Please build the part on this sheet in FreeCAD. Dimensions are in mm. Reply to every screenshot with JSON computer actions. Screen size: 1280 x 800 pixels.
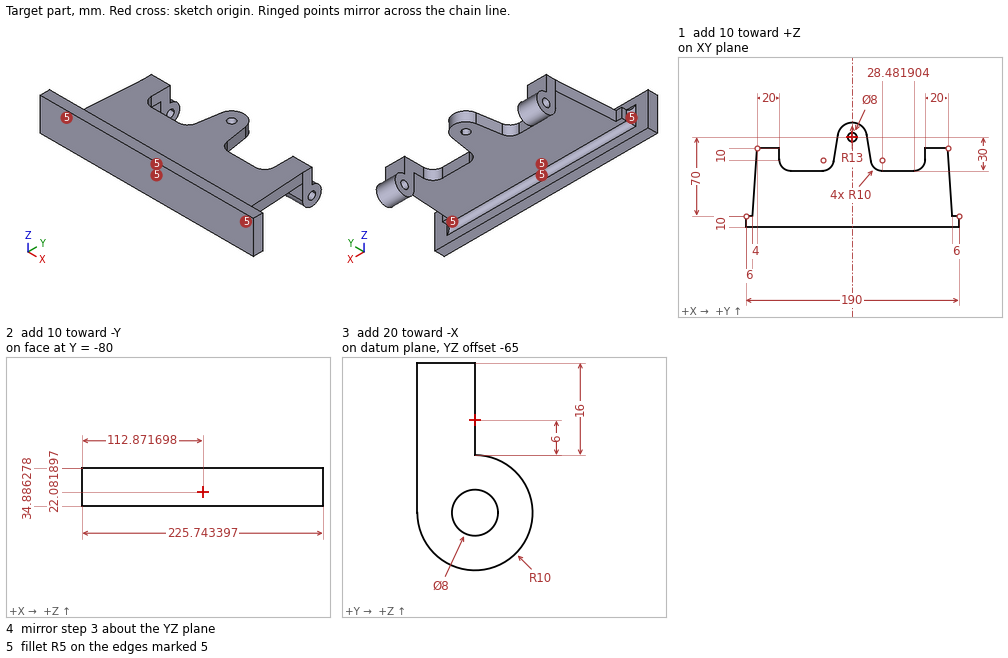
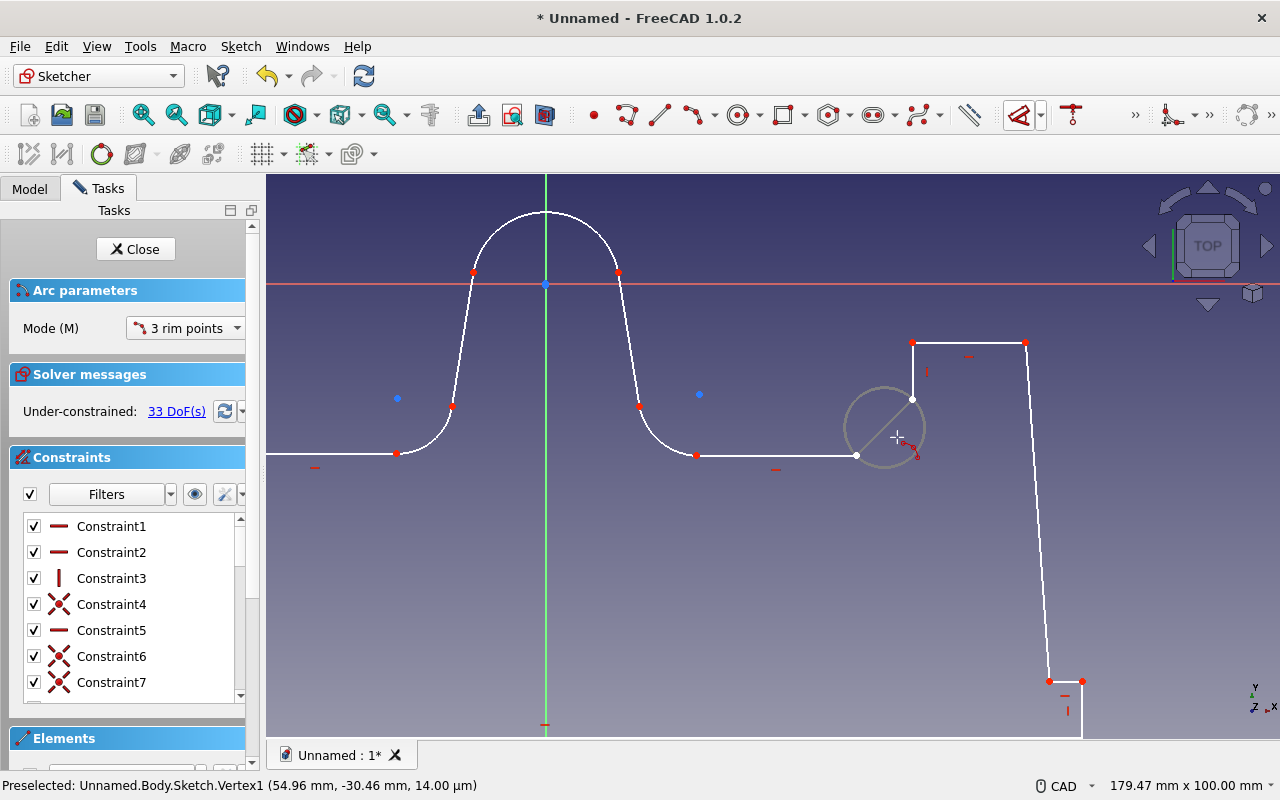
{"action": "left_click", "coordinate": [897, 437]}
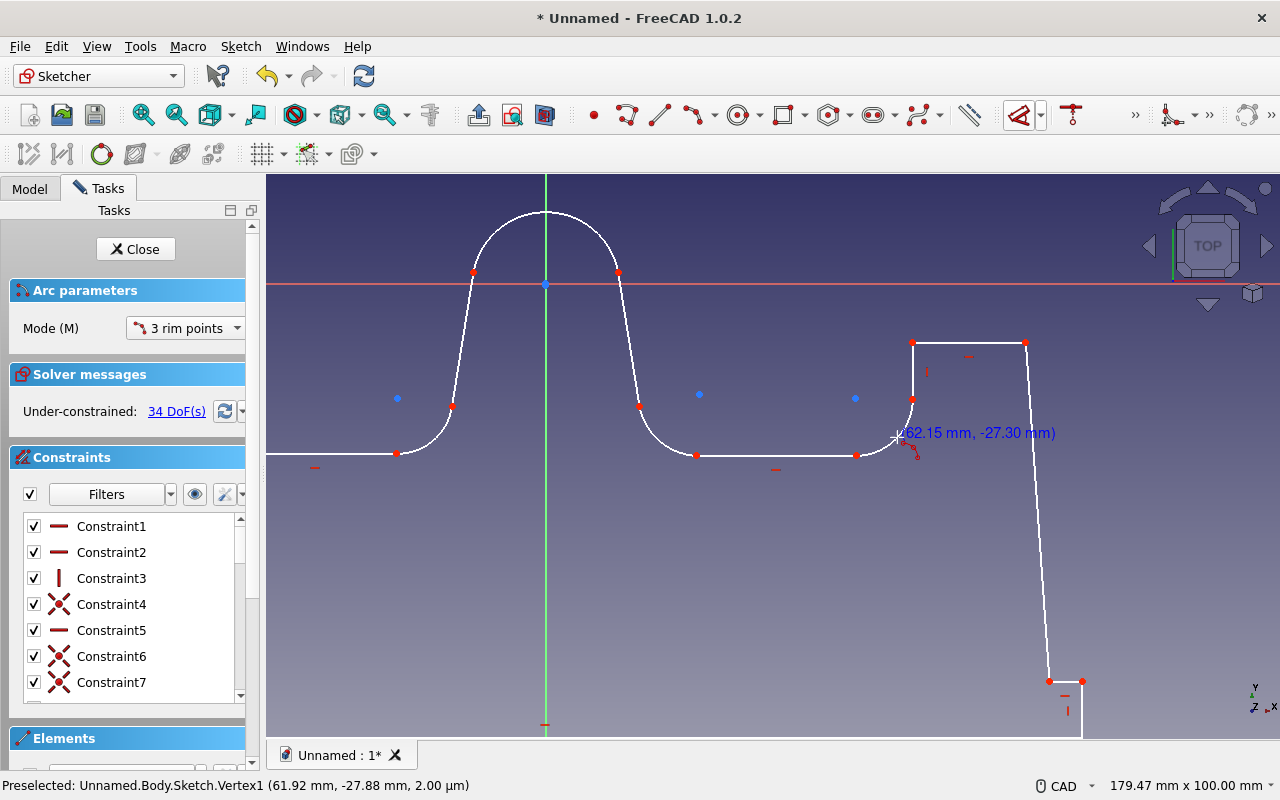
{"action": "left_click", "coordinate": [738, 116]}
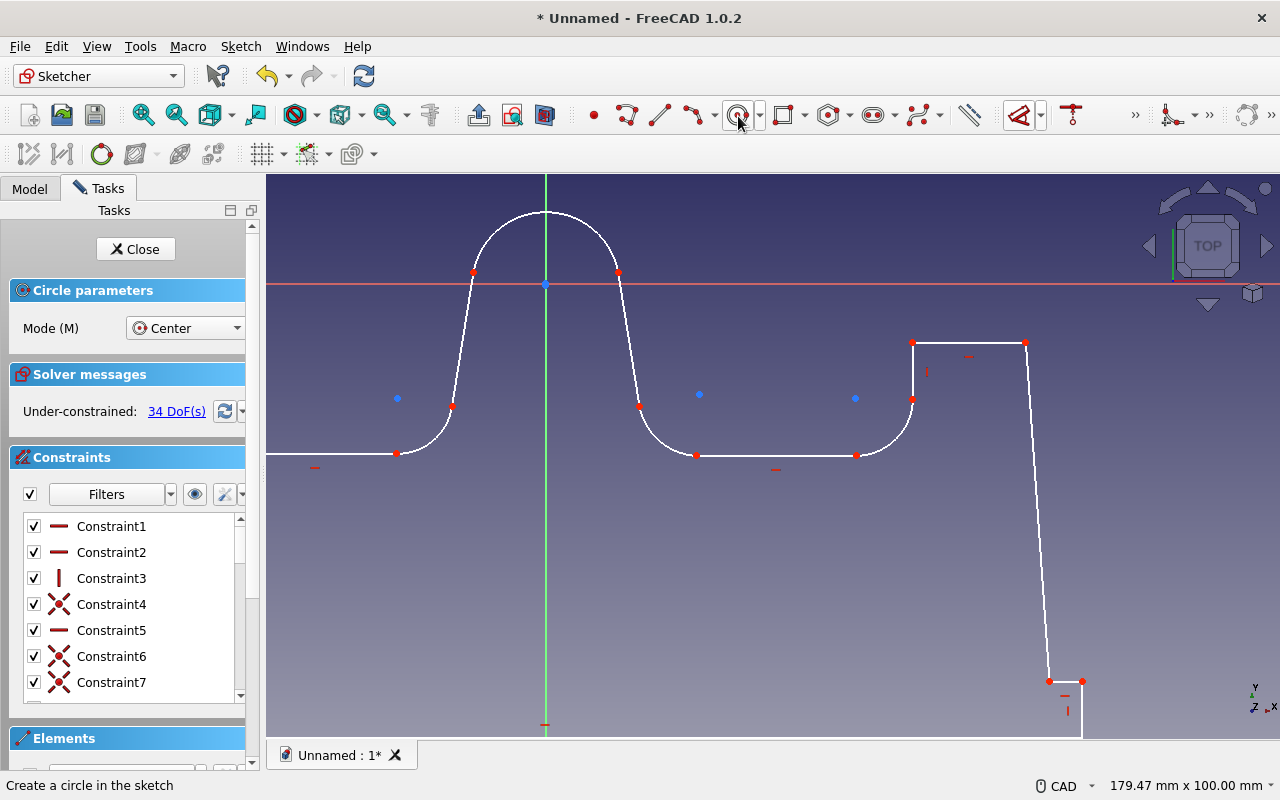
{"action": "left_click", "coordinate": [546, 284]}
{"action": "left_click", "coordinate": [562, 268]}
{"action": "key", "text": "Escape"}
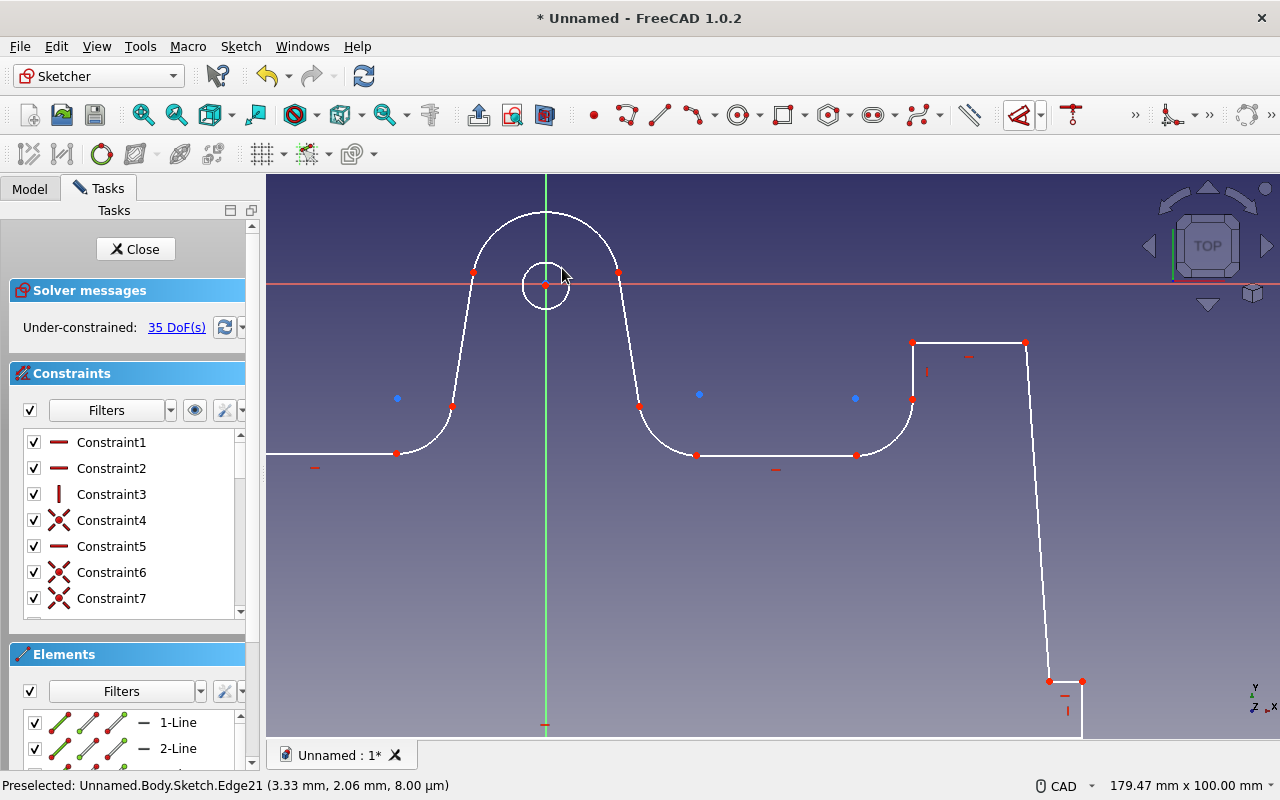
{"action": "left_click", "coordinate": [808, 456]}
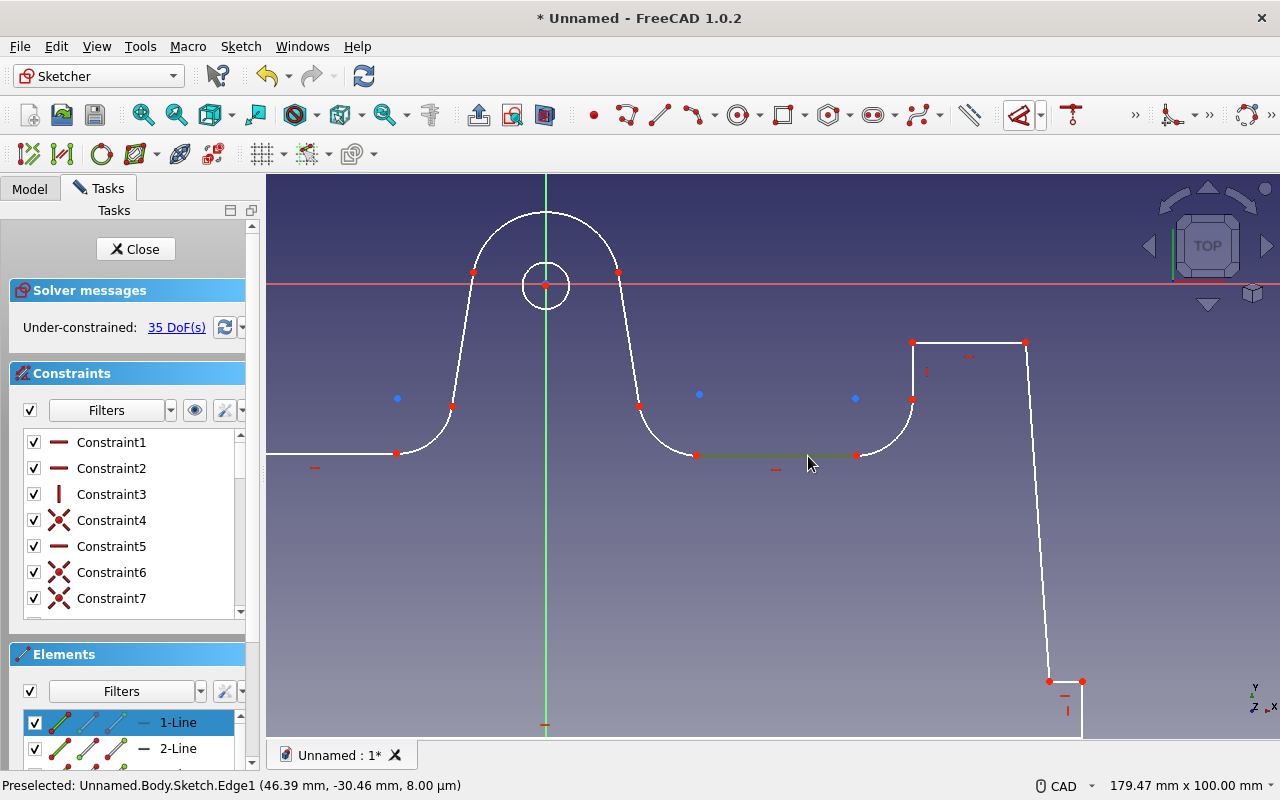
{"action": "left_click", "coordinate": [649, 429]}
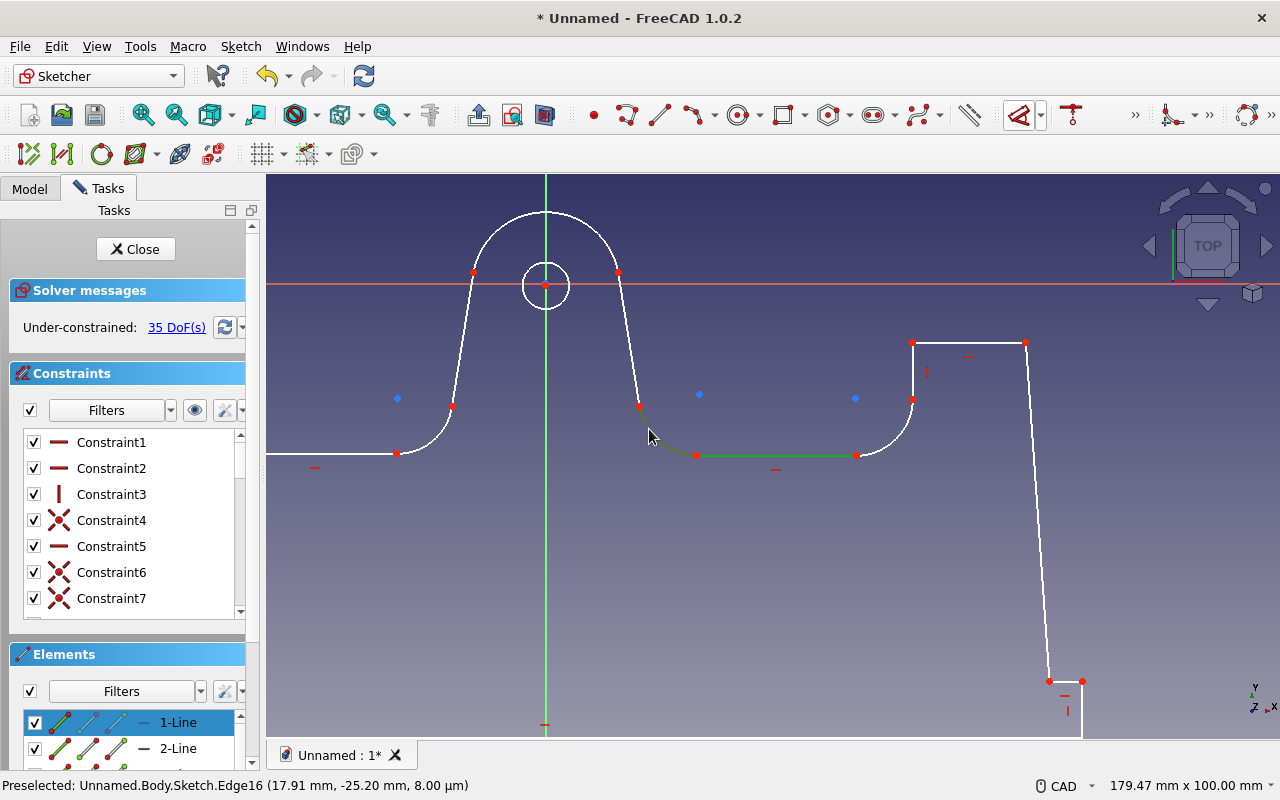
{"action": "key", "text": "t"}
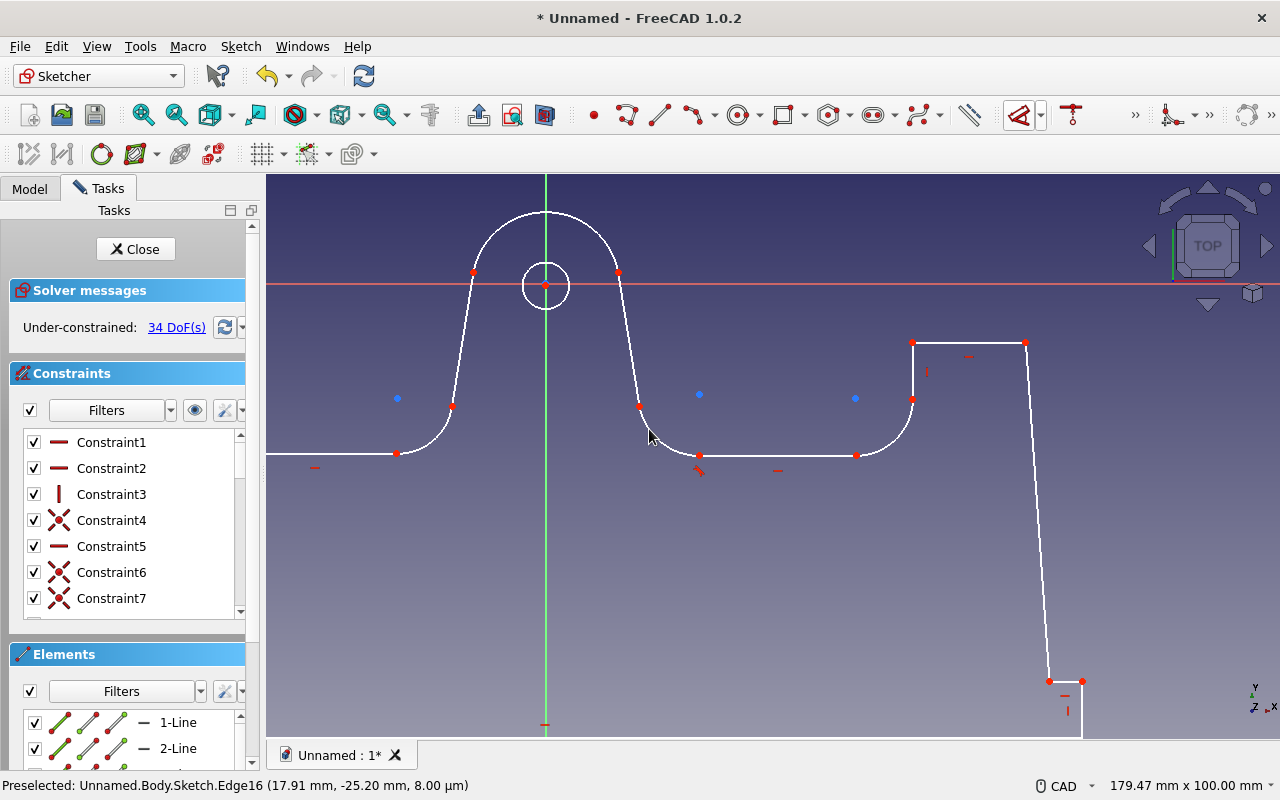
{"action": "left_click", "coordinate": [809, 456]}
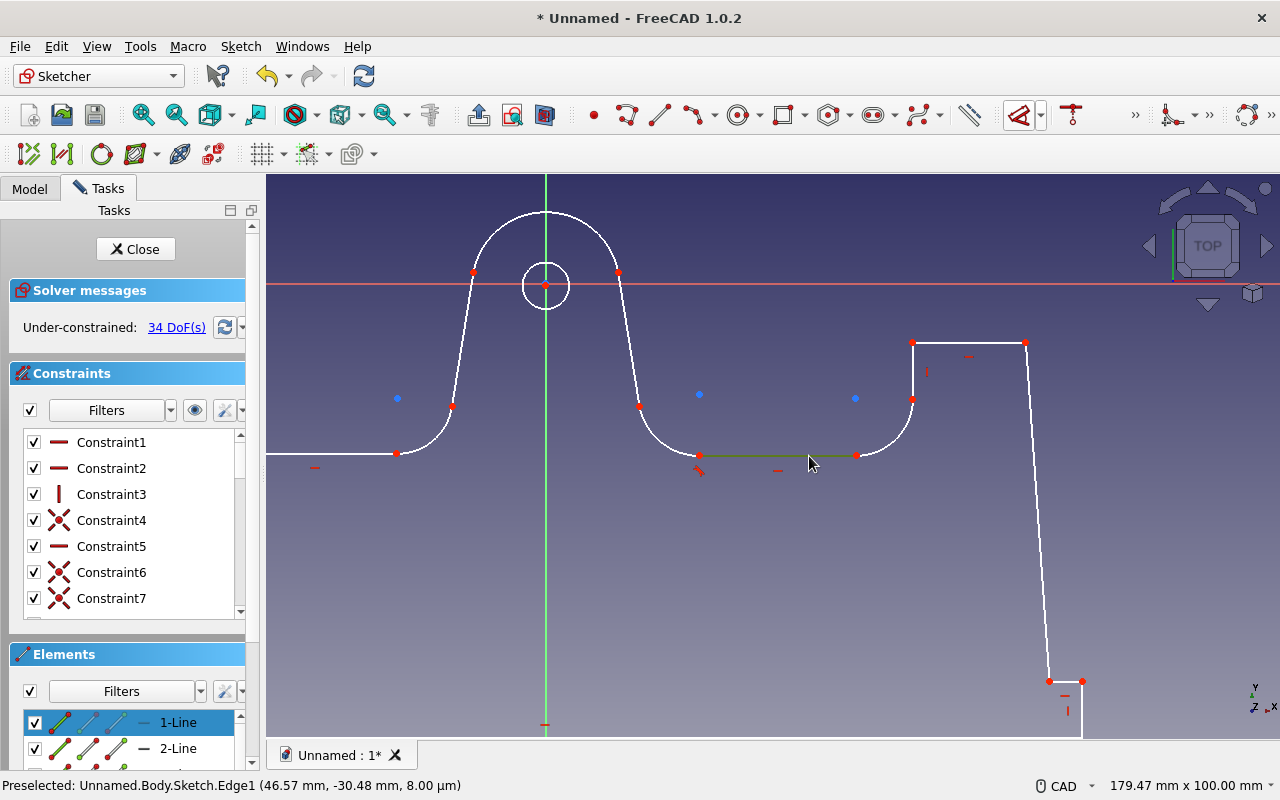
{"action": "left_click", "coordinate": [882, 449]}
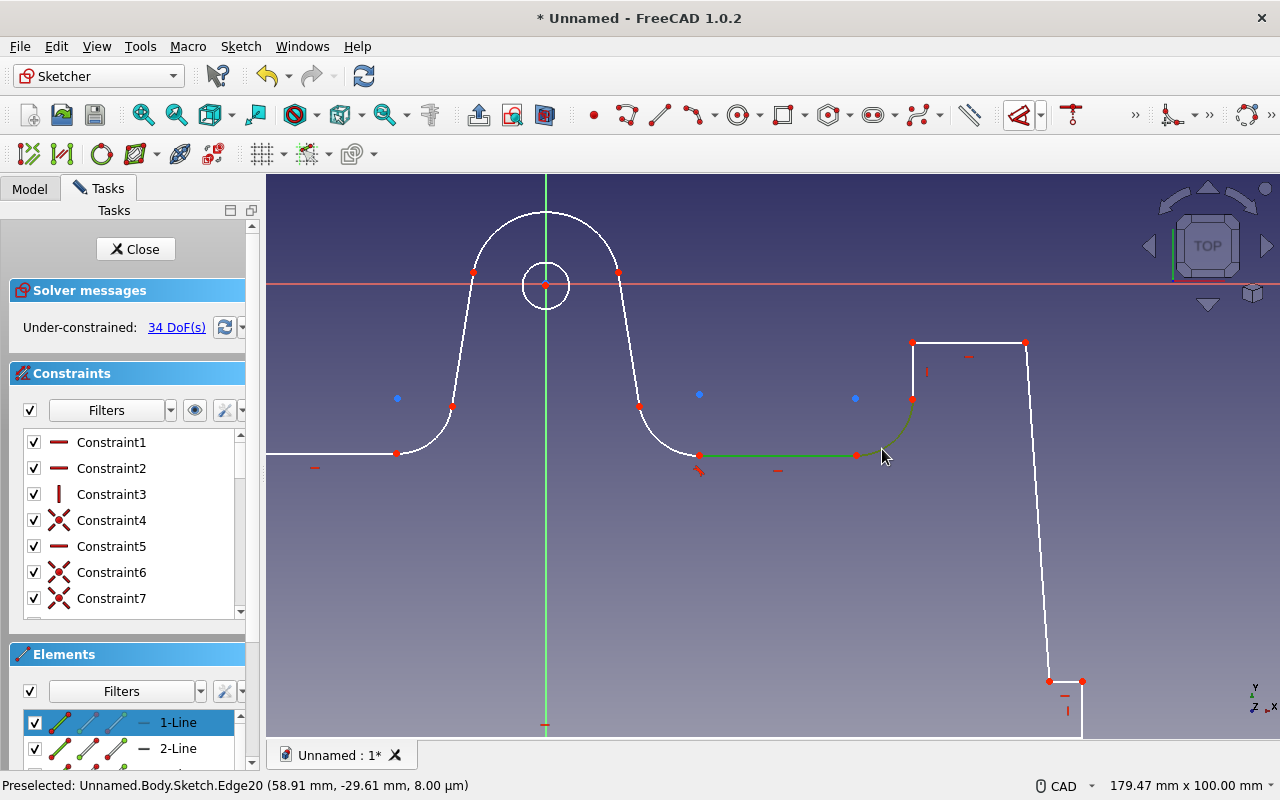
{"action": "key", "text": "t"}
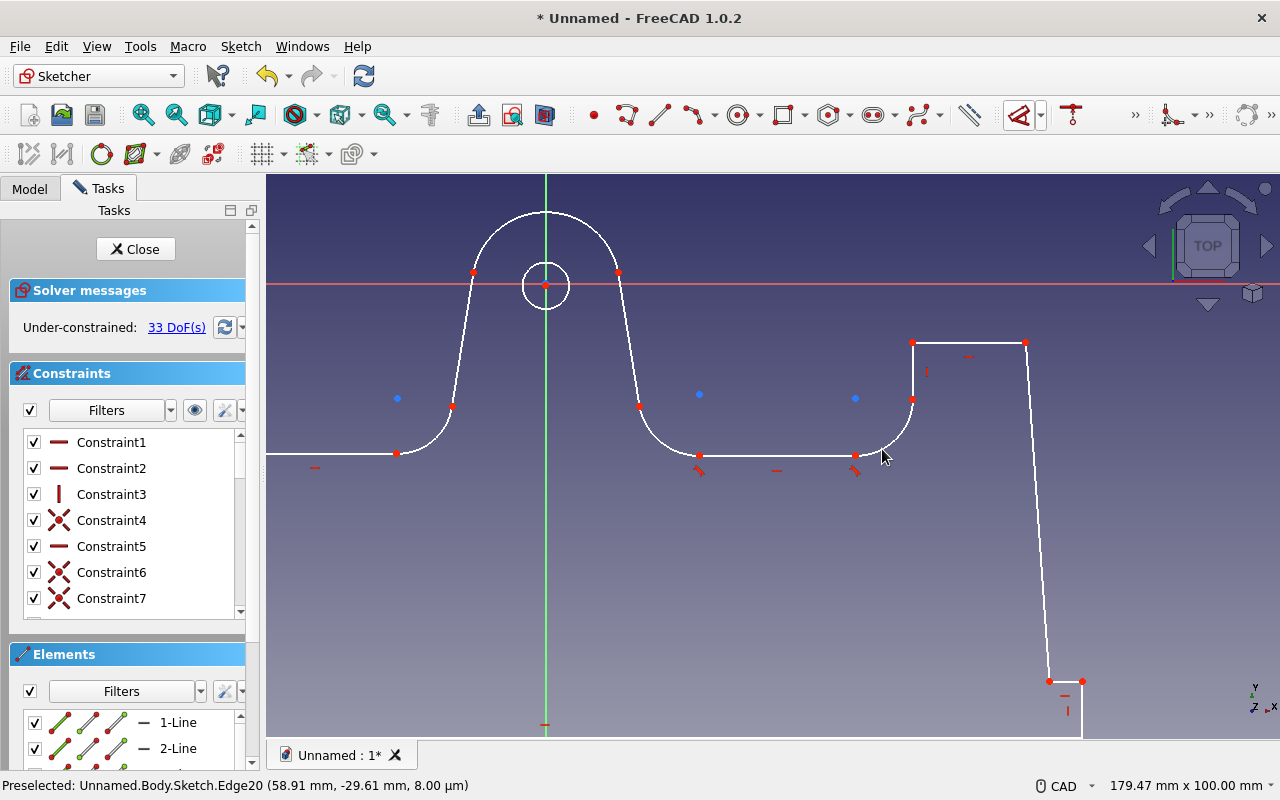
{"action": "left_click", "coordinate": [633, 367]}